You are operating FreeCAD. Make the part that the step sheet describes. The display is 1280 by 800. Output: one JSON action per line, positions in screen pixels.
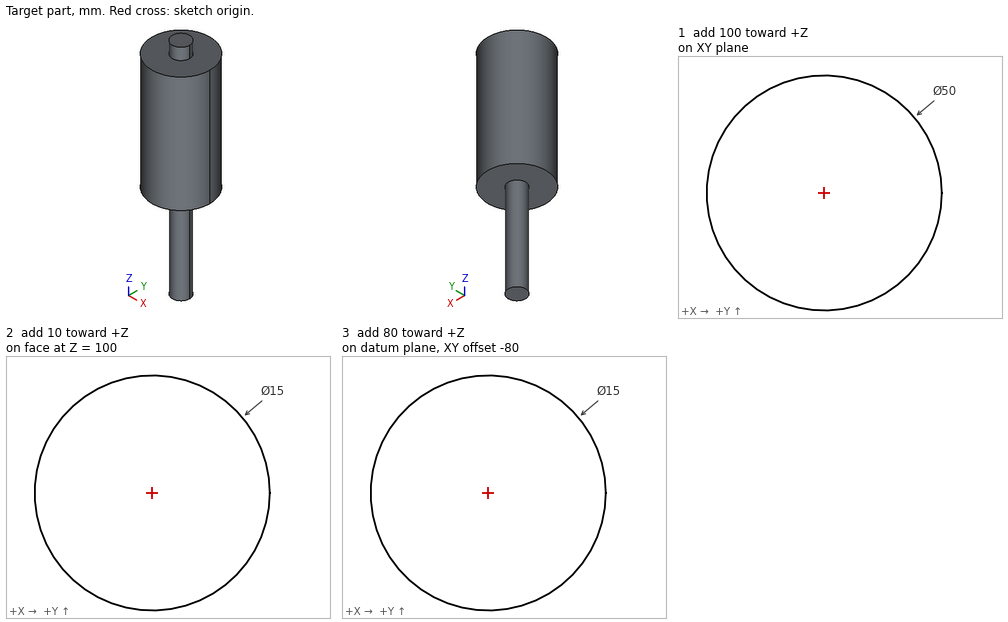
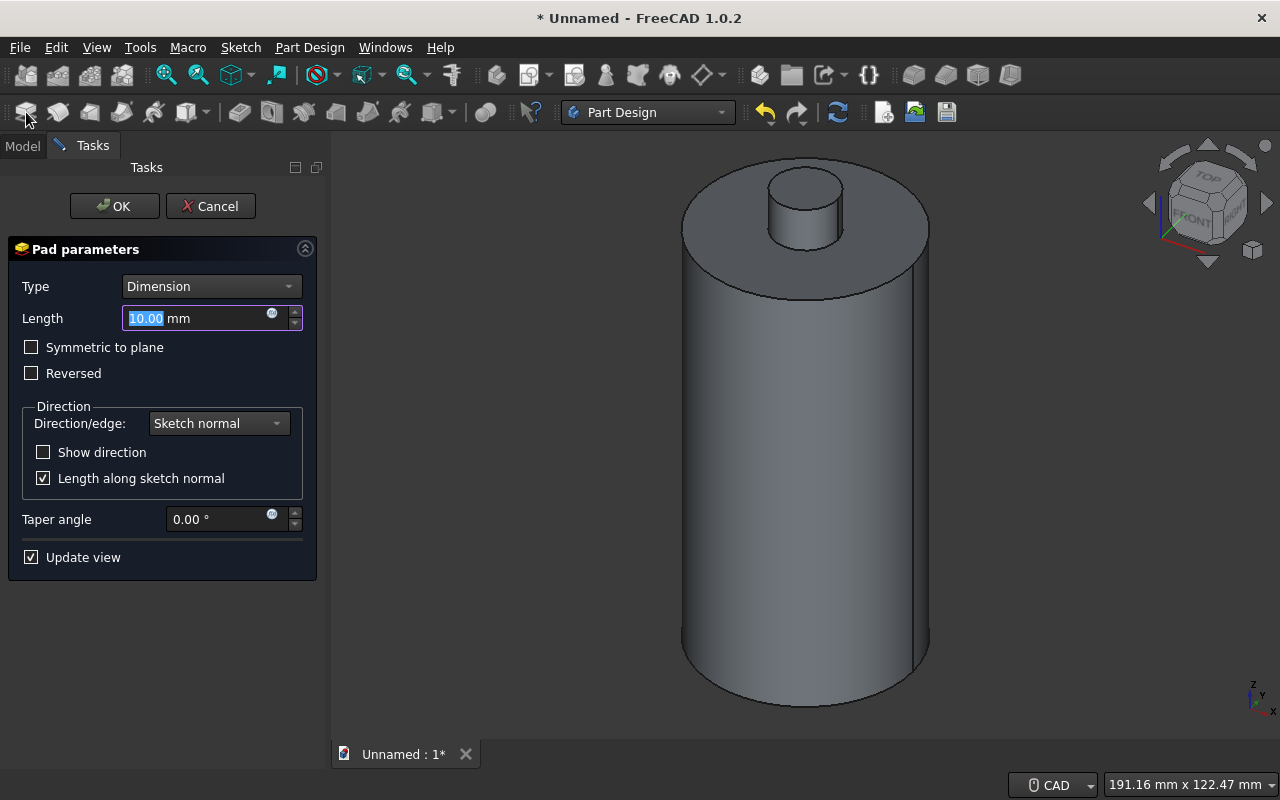
{"action": "type", "text": "10"}
{"action": "key", "text": "Tab"}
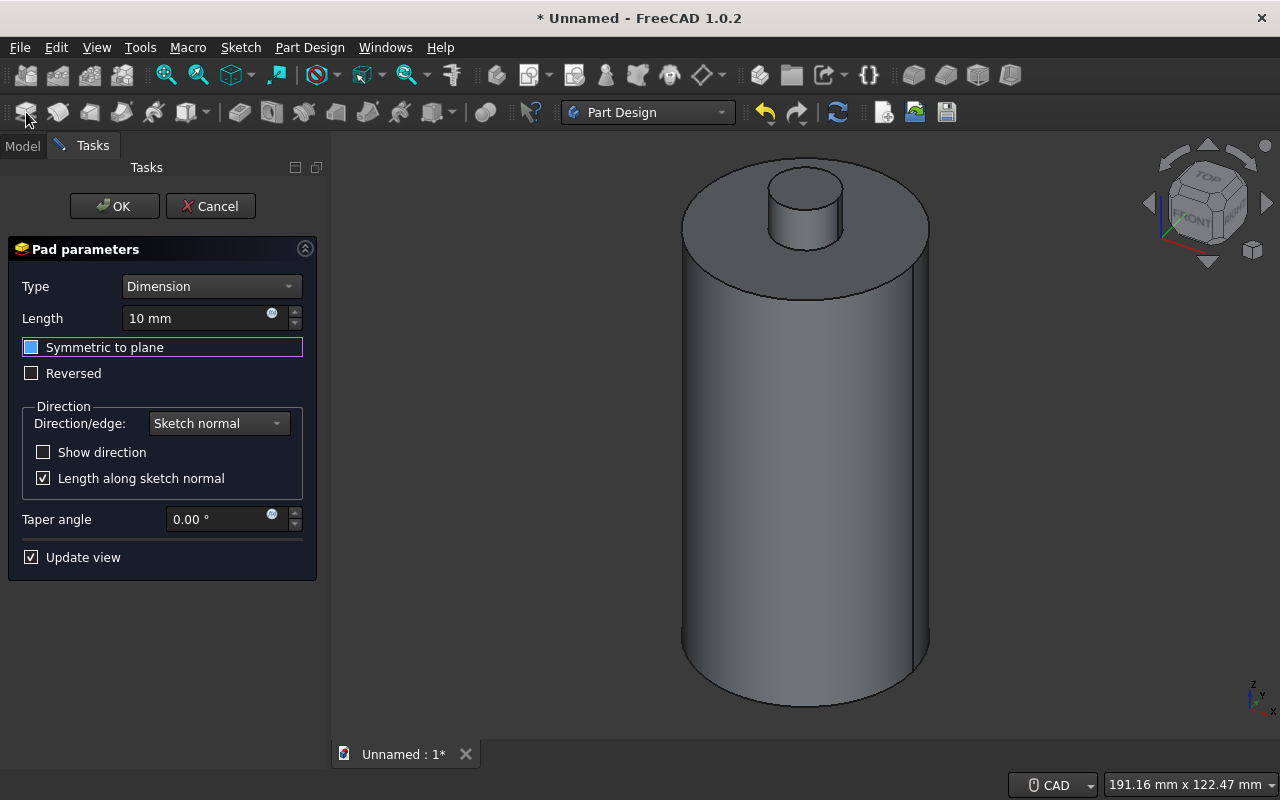
{"action": "left_click", "coordinate": [115, 206]}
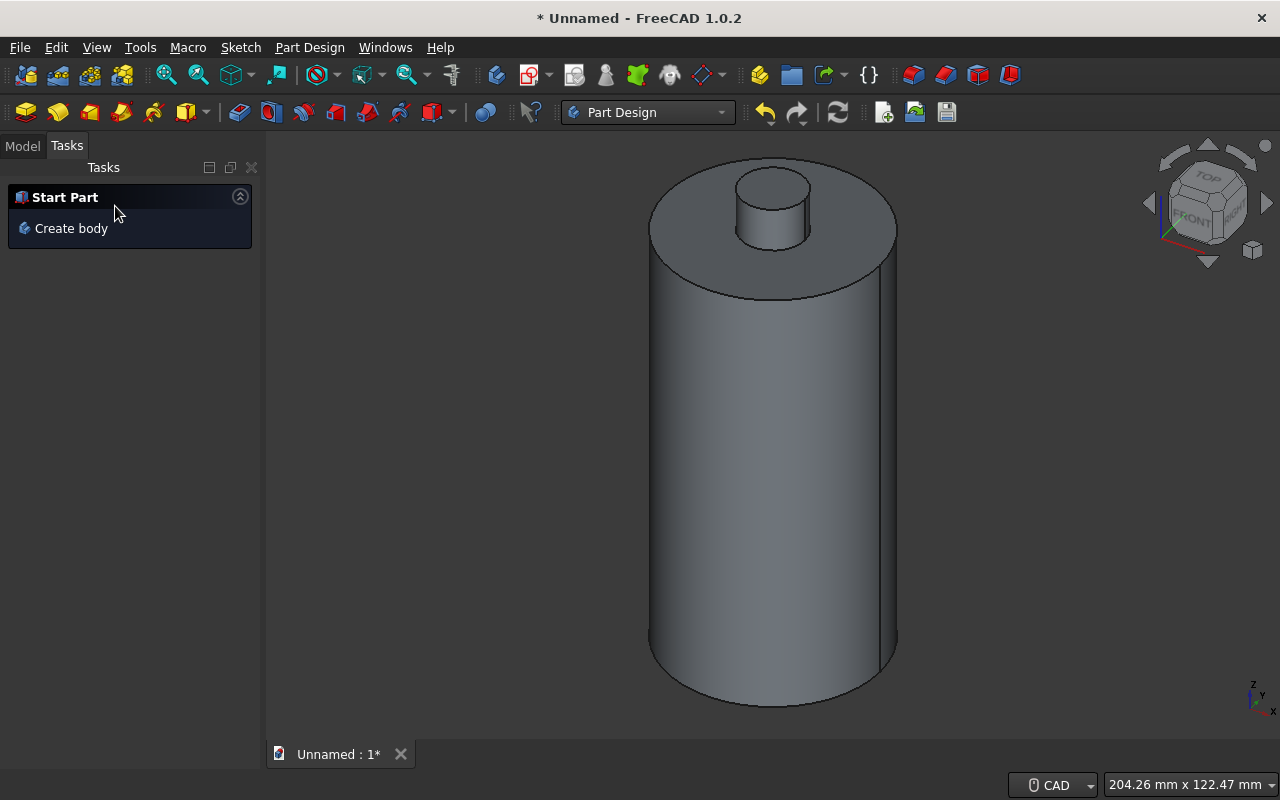
{"action": "left_click", "coordinate": [168, 76]}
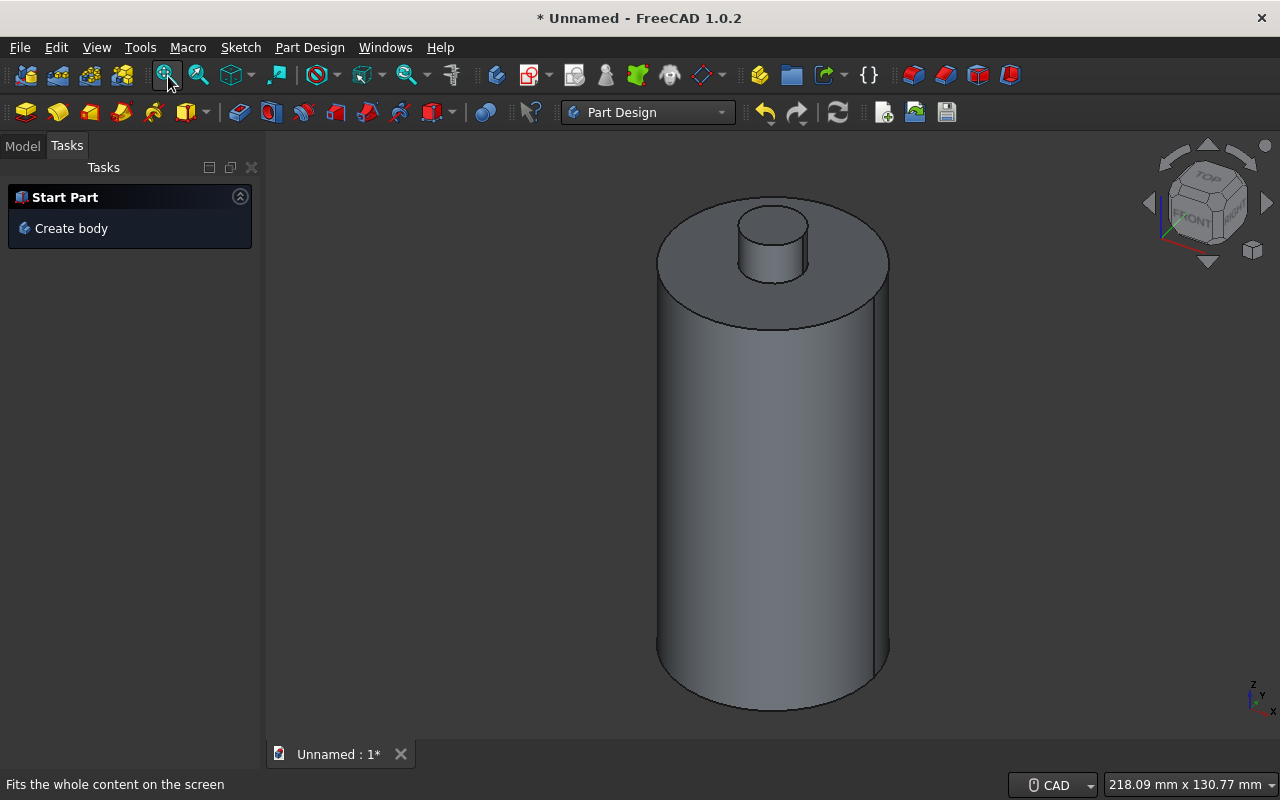
{"action": "left_click", "coordinate": [23, 145]}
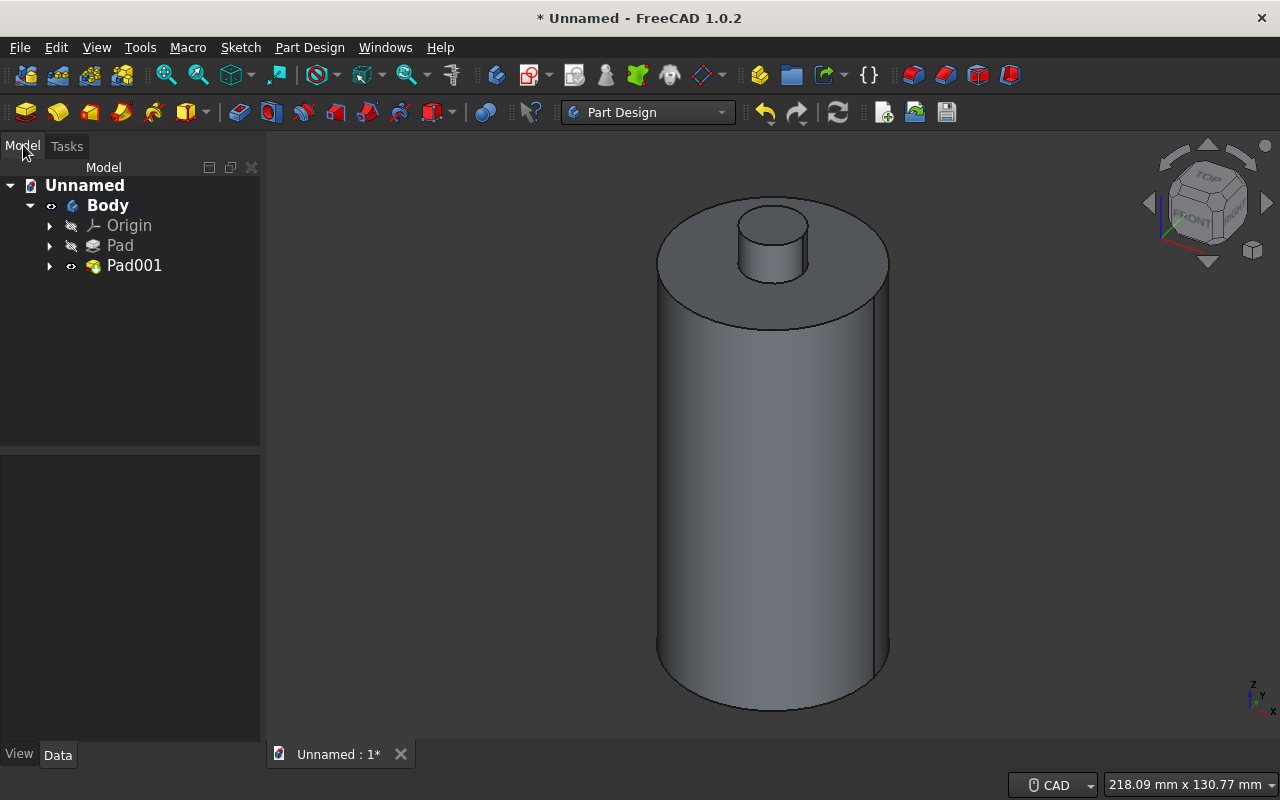
{"action": "left_click", "coordinate": [50, 226]}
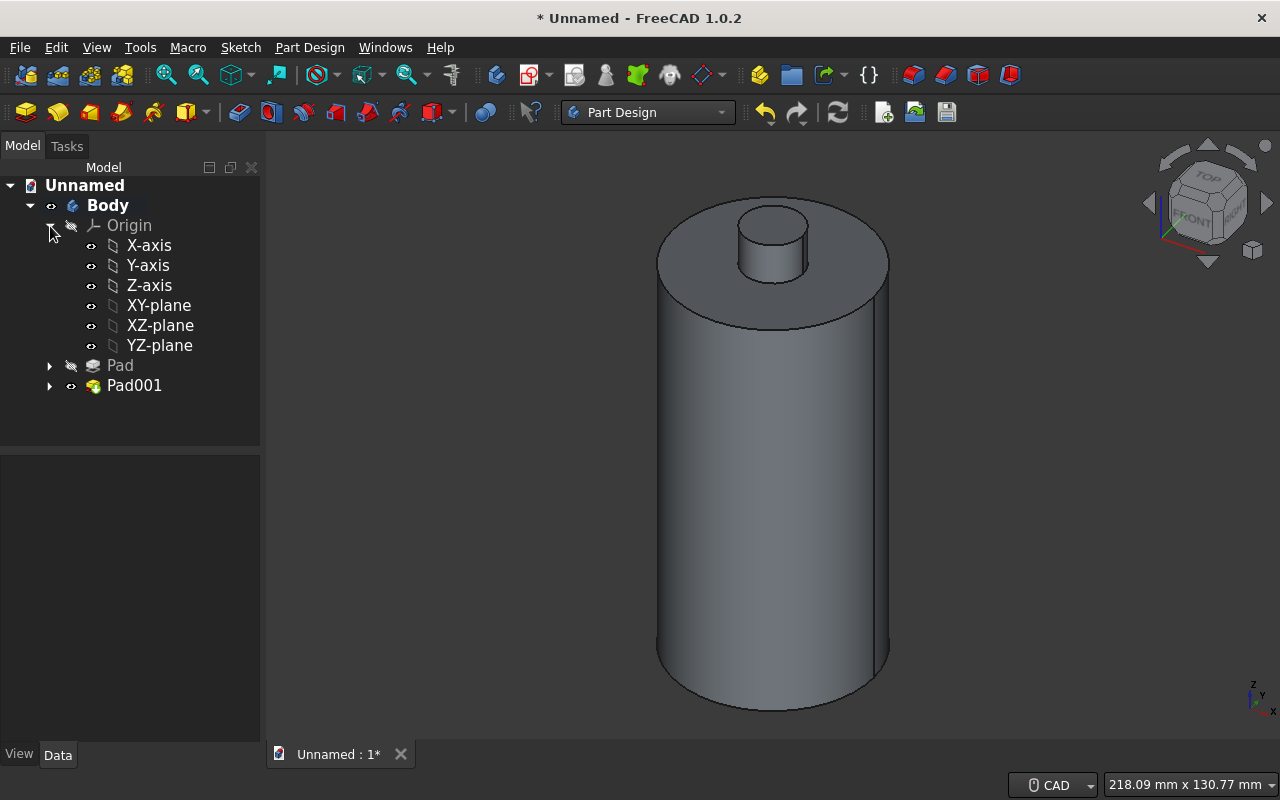
{"action": "left_click", "coordinate": [136, 306]}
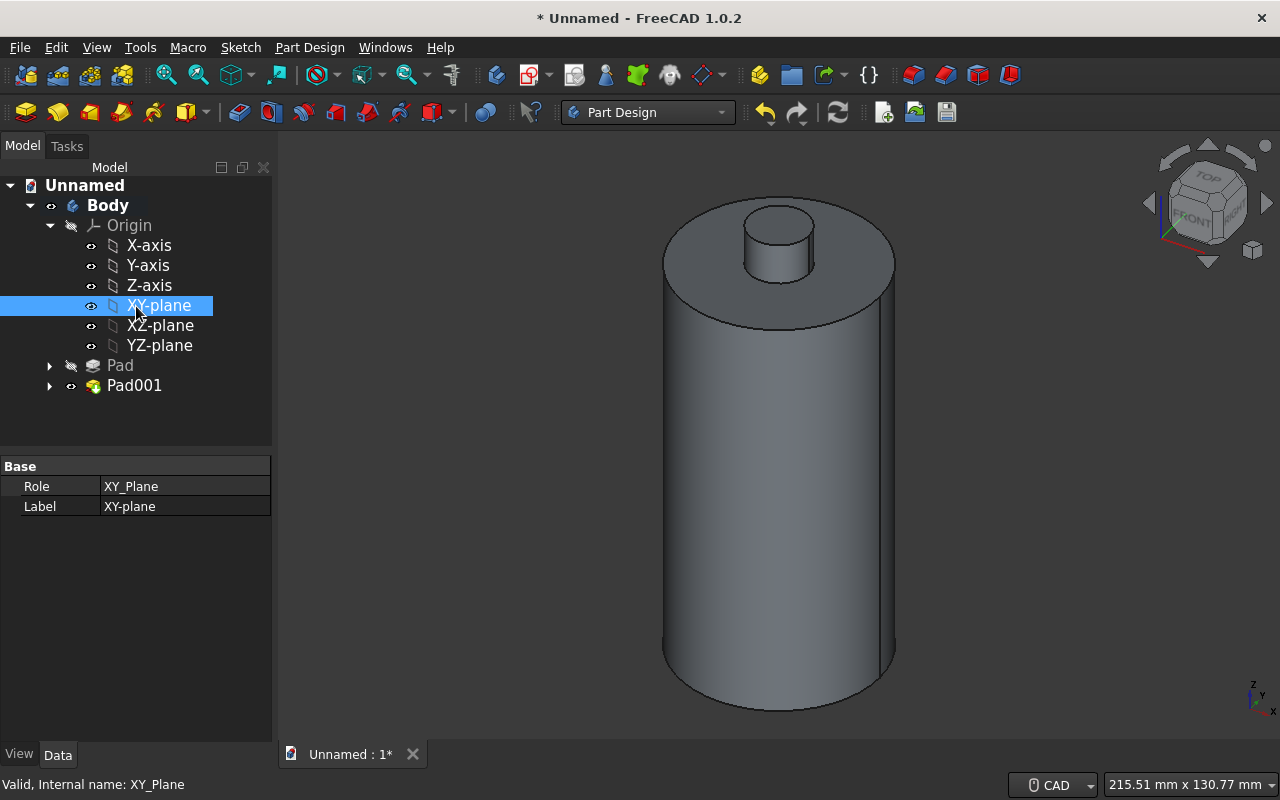
{"action": "left_click", "coordinate": [702, 76]}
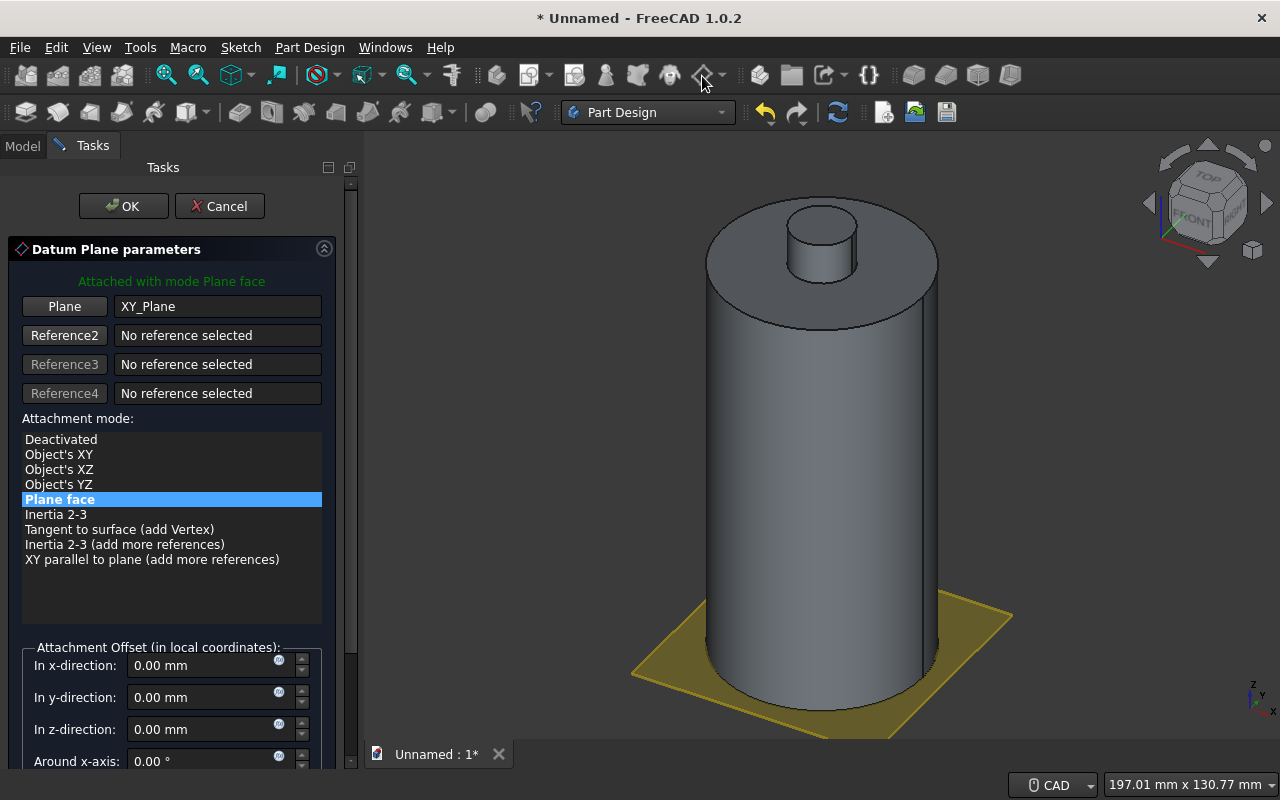
{"action": "triple_click", "coordinate": [210, 729]}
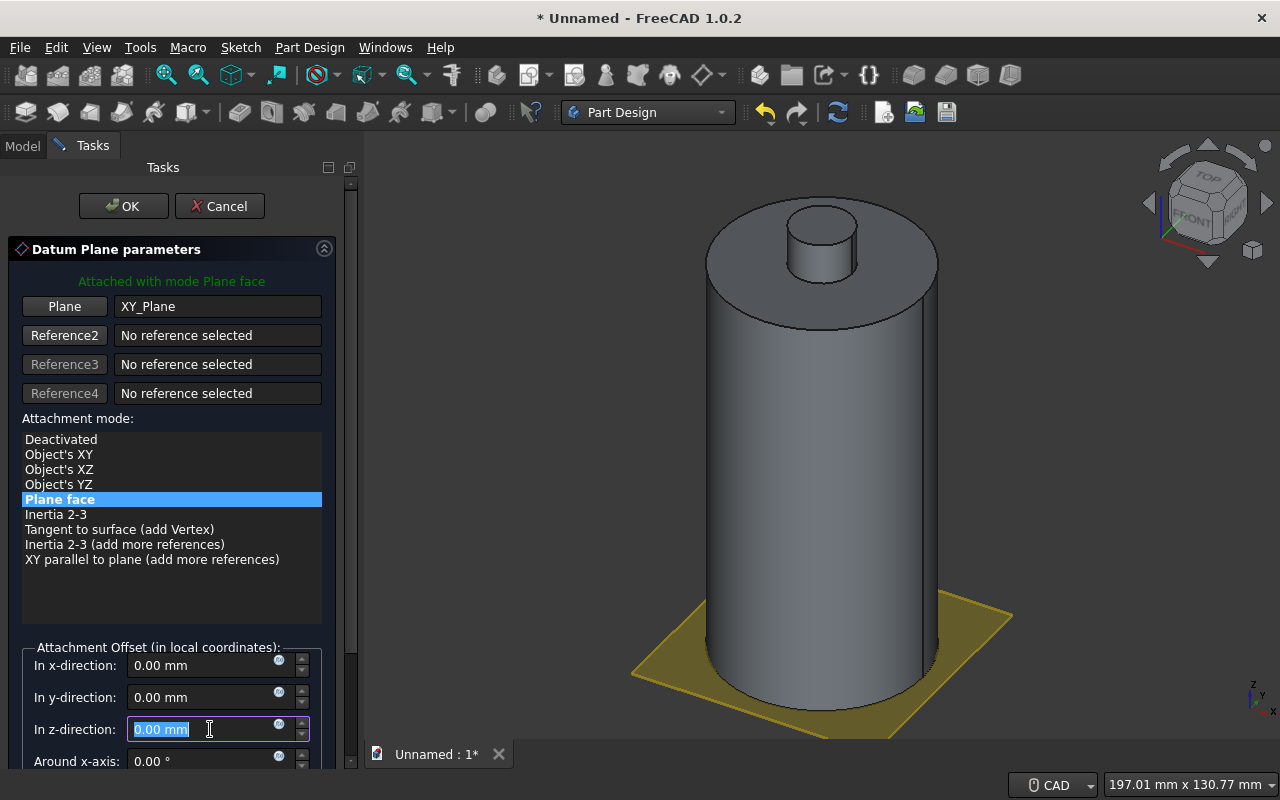
{"action": "type", "text": "-80"}
{"action": "key", "text": "Tab"}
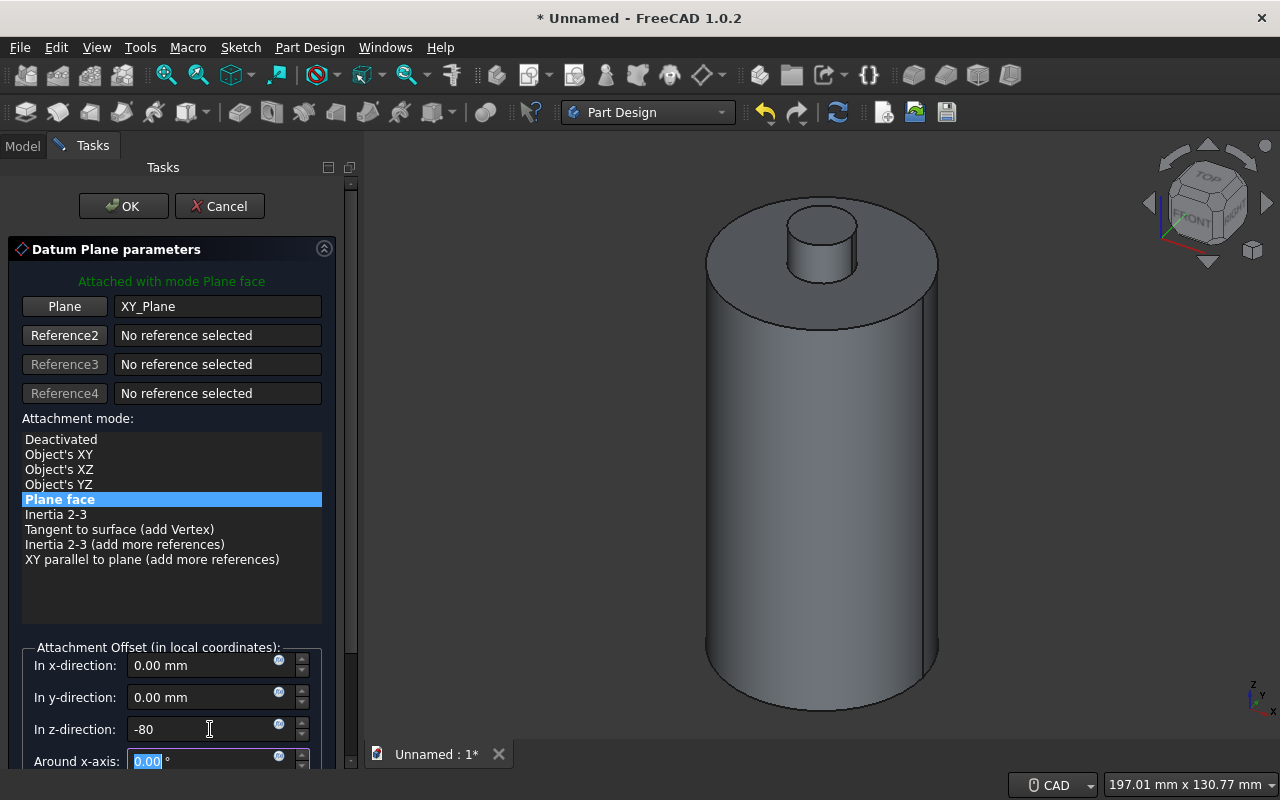
{"action": "left_click", "coordinate": [124, 206]}